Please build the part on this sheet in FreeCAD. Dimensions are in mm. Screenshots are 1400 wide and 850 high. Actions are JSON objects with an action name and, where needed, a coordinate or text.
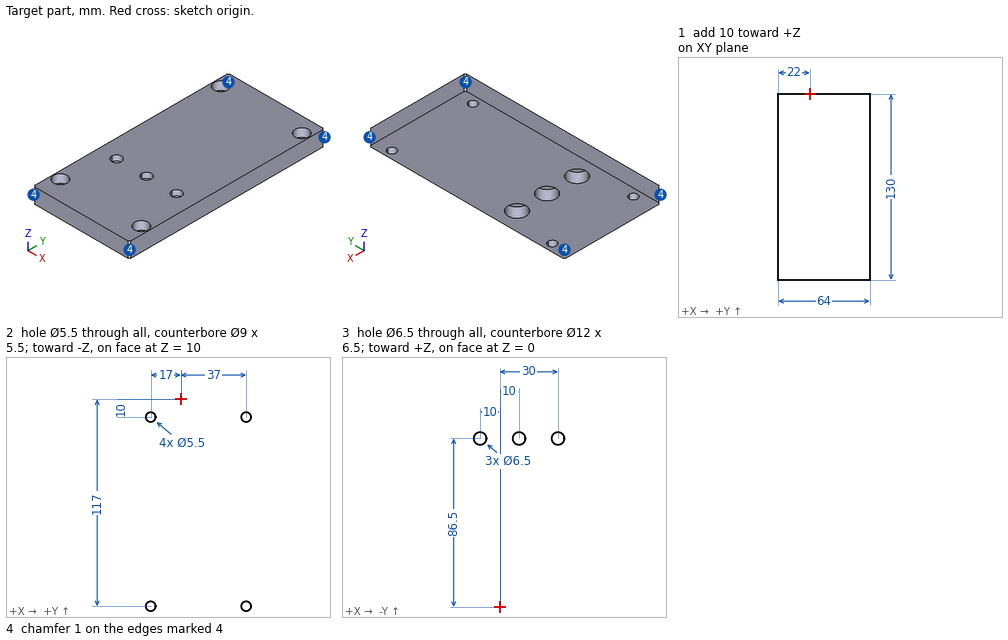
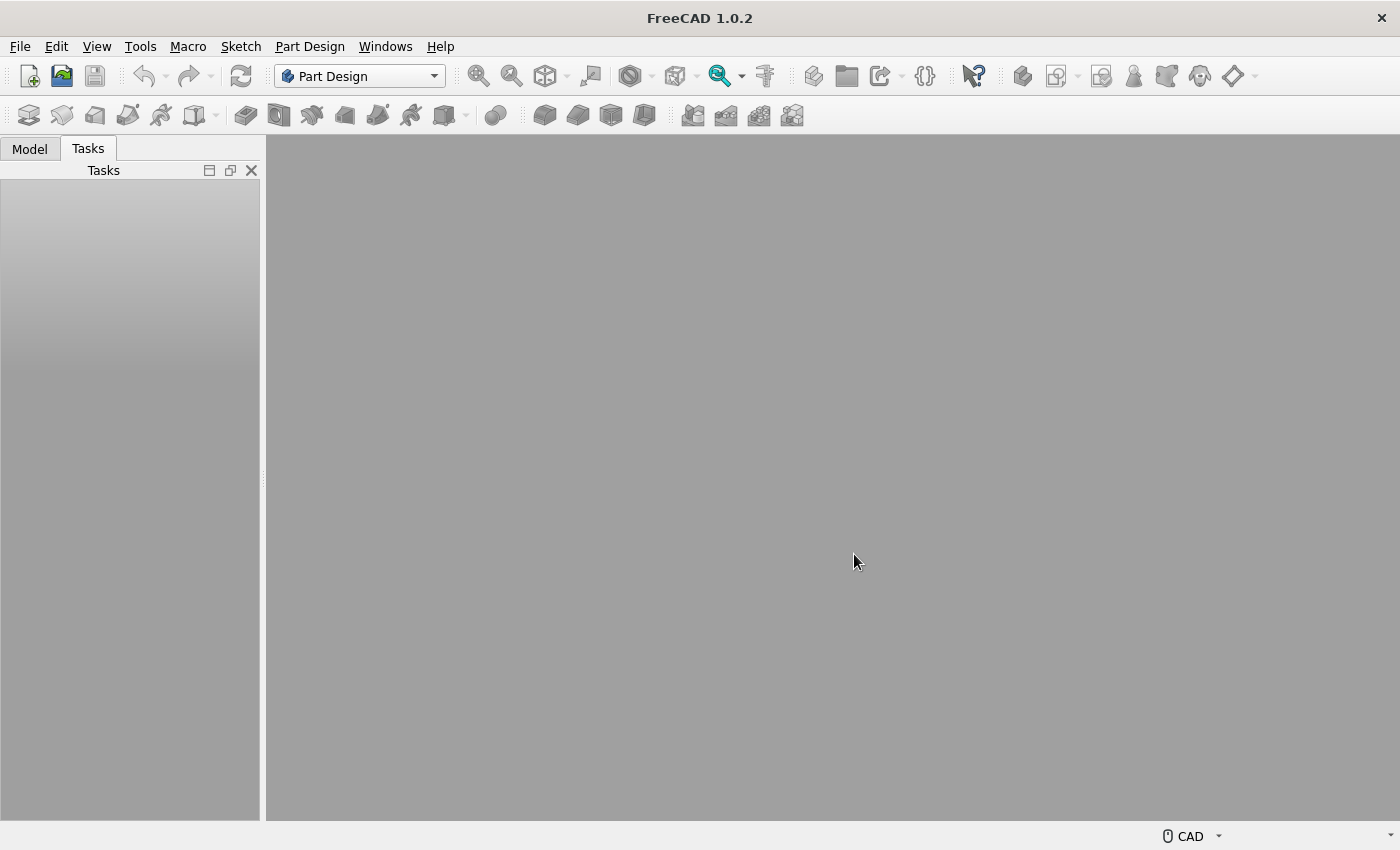
{"action": "left_click", "coordinate": [29, 76]}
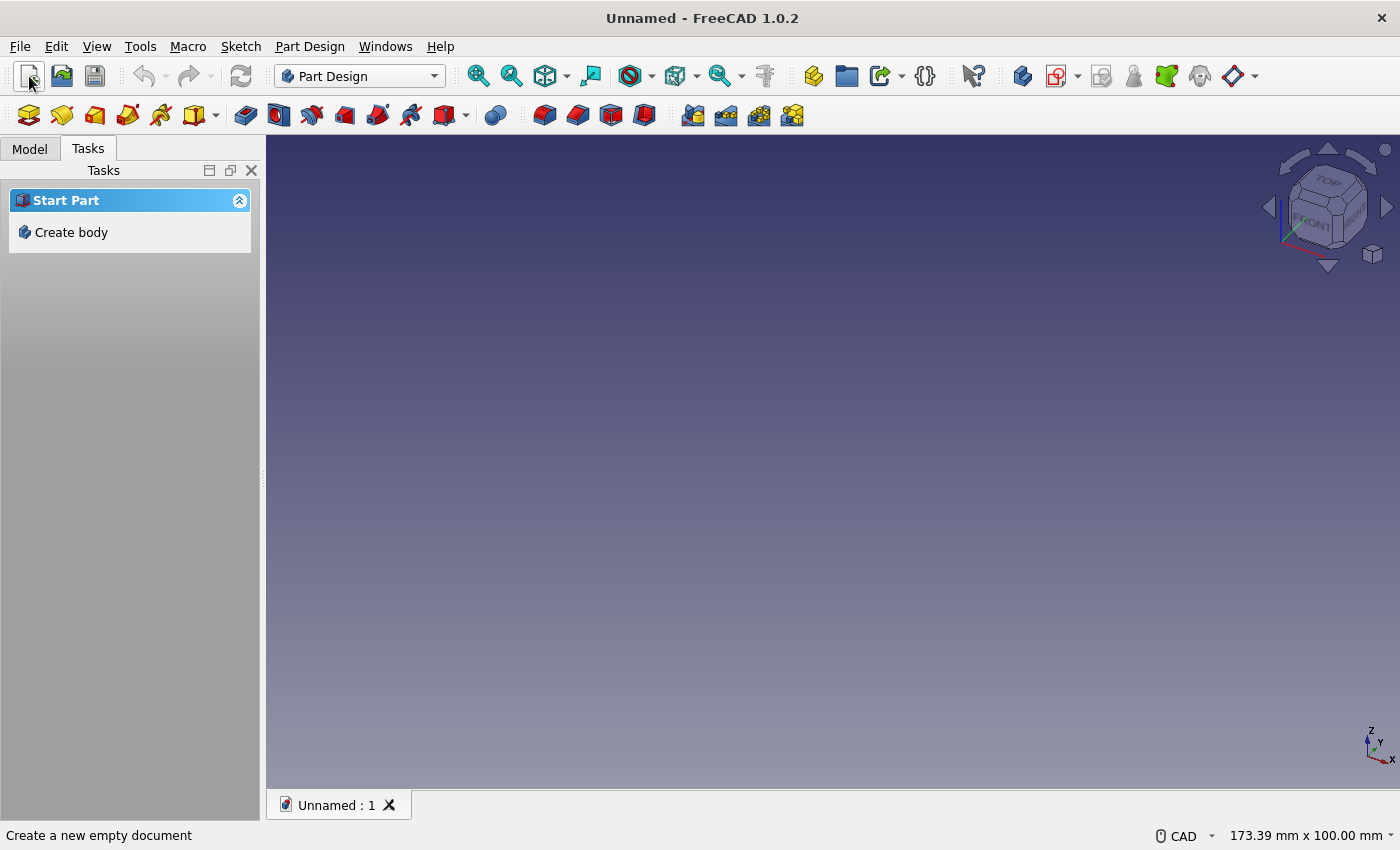
{"action": "left_click", "coordinate": [1056, 76]}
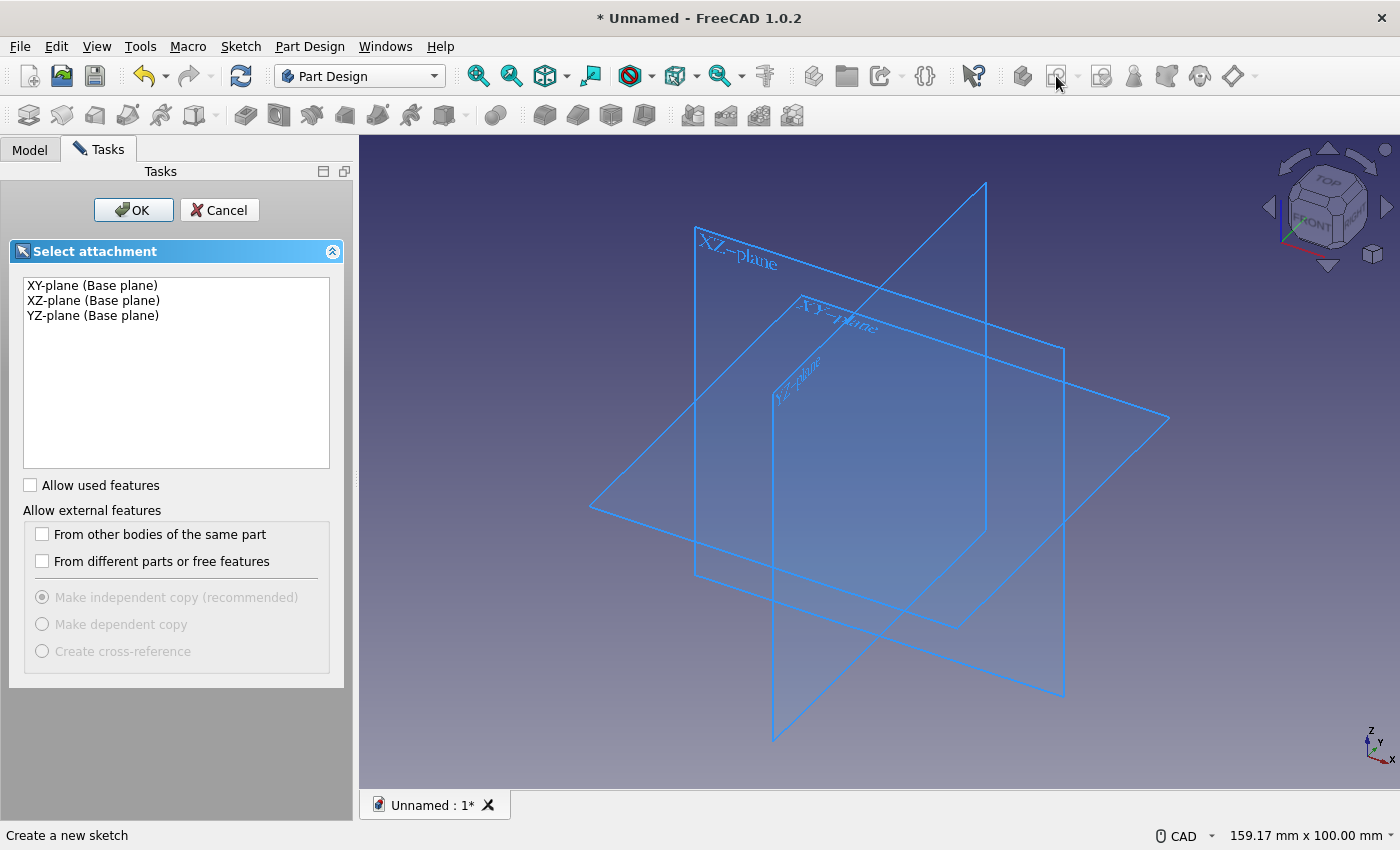
{"action": "left_click", "coordinate": [84, 286]}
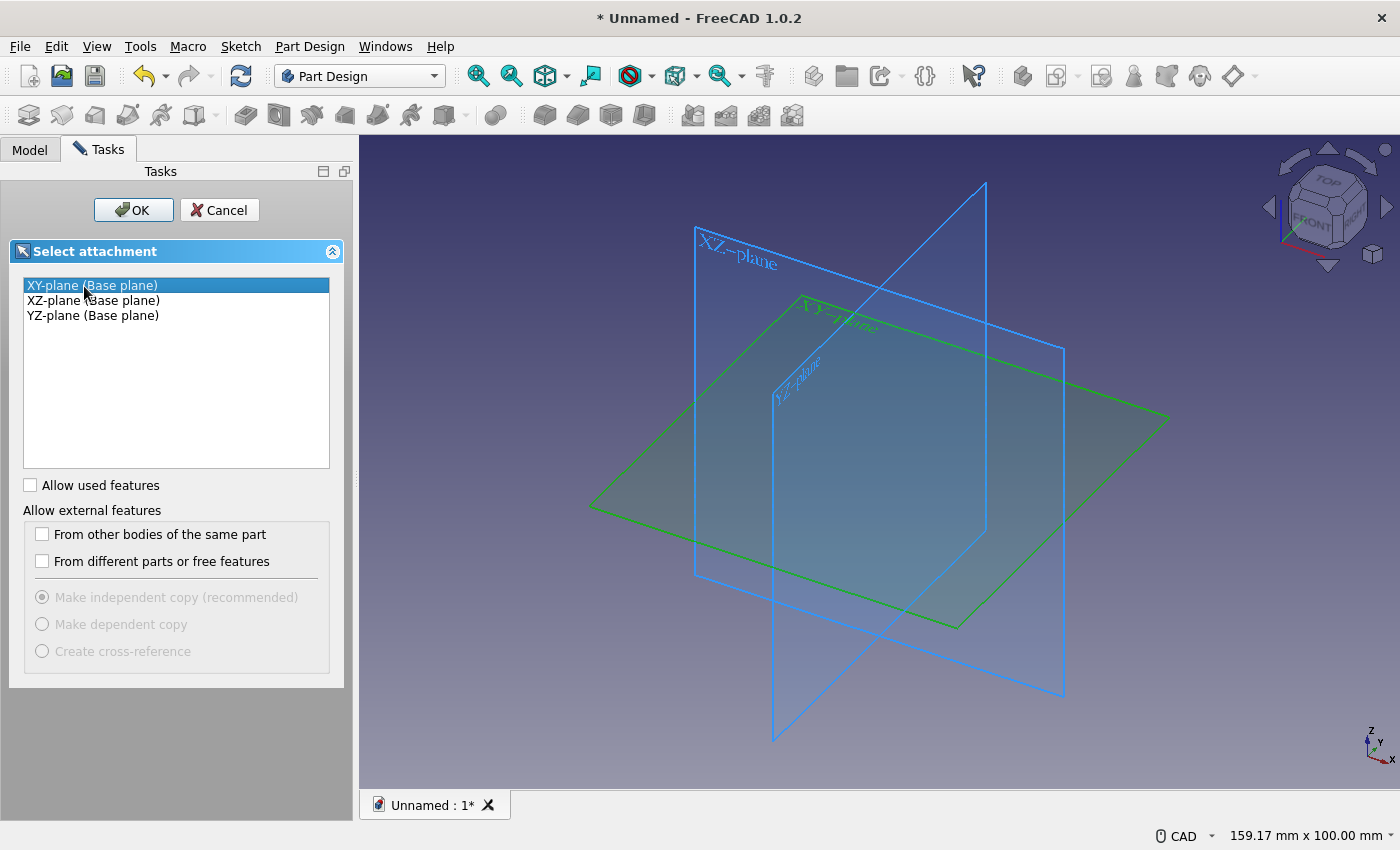
{"action": "left_click", "coordinate": [134, 210]}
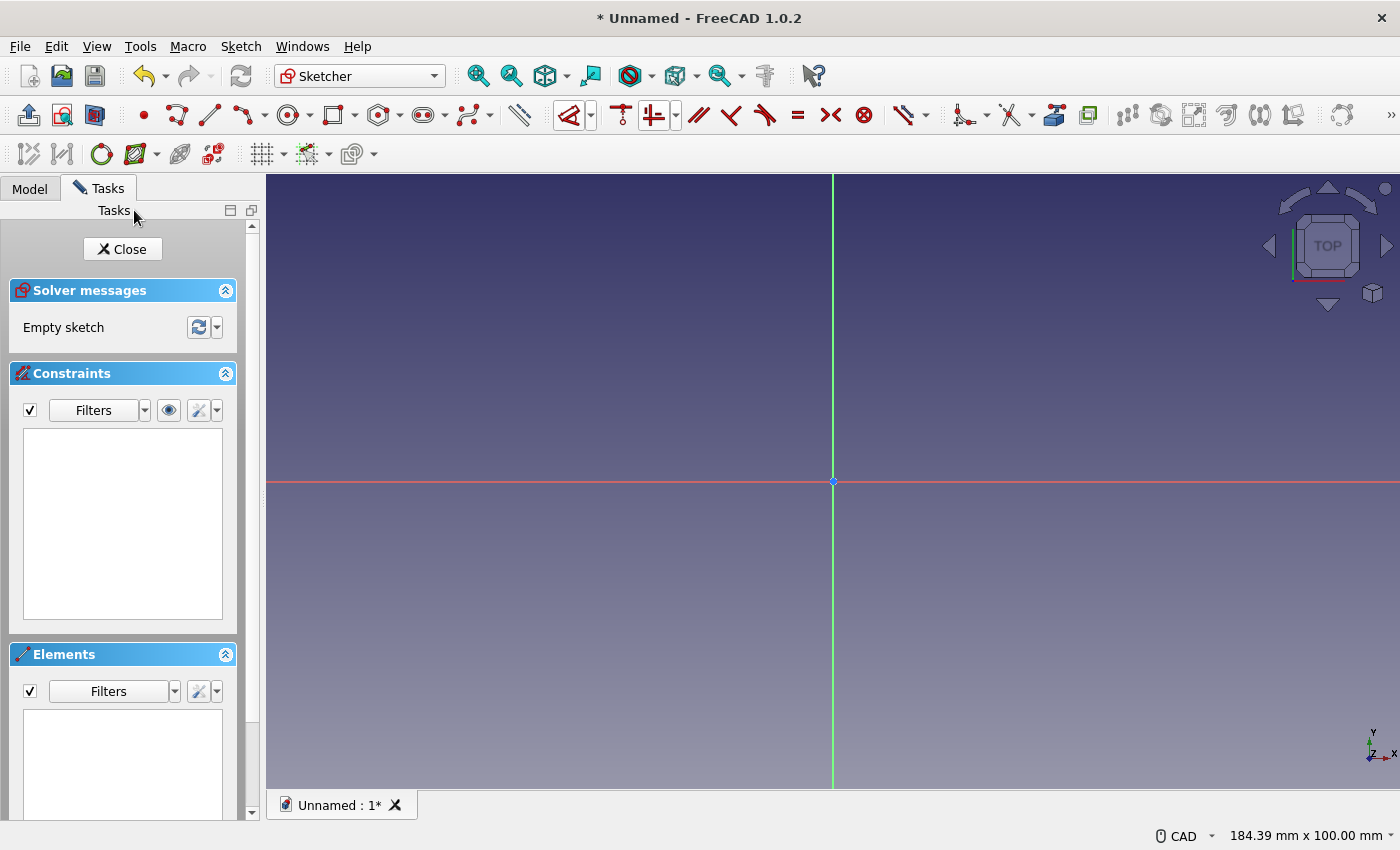
{"action": "scroll", "coordinate": [658, 202], "scroll_direction": "down", "scroll_amount": 4}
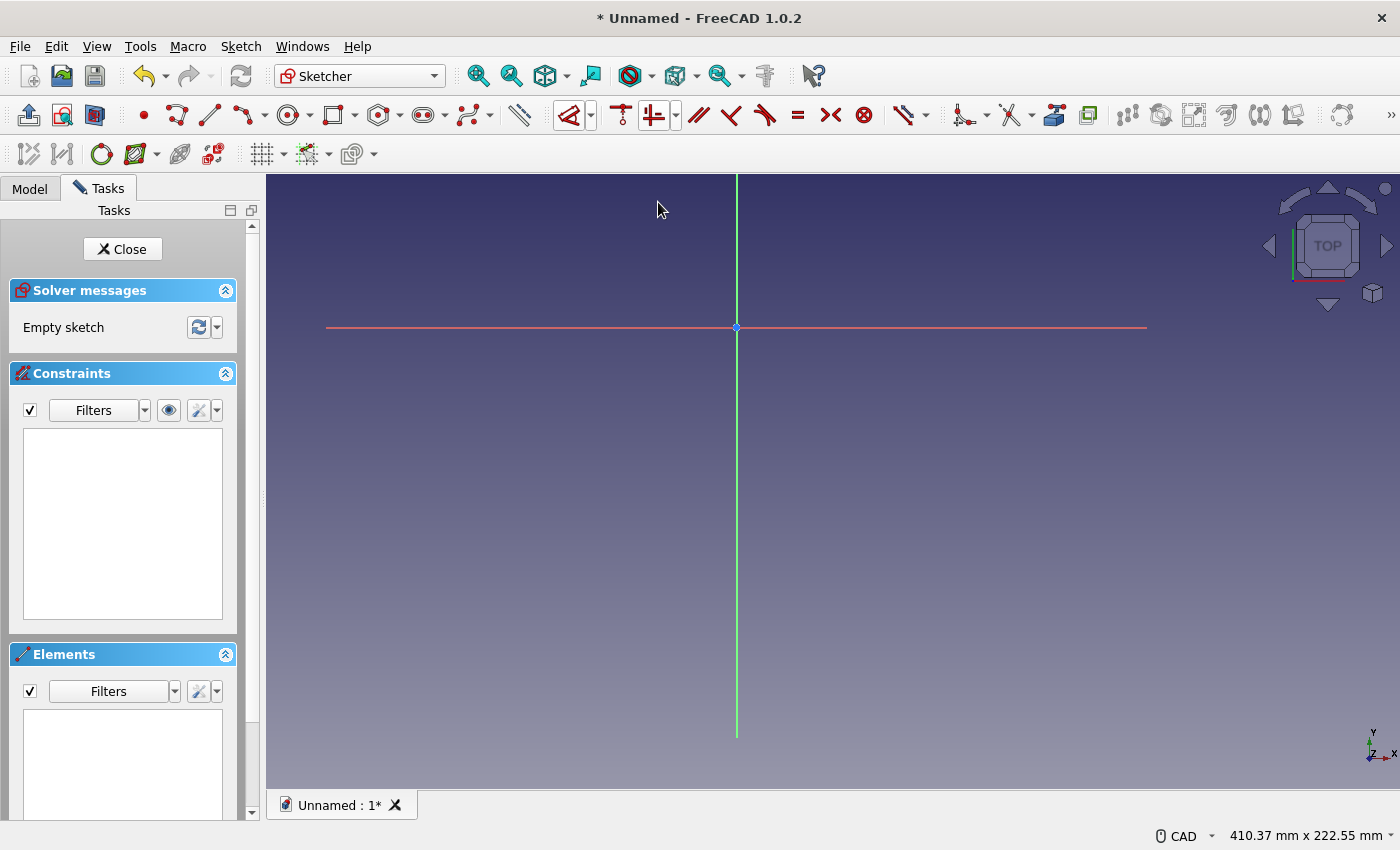
{"action": "left_click", "coordinate": [332, 116]}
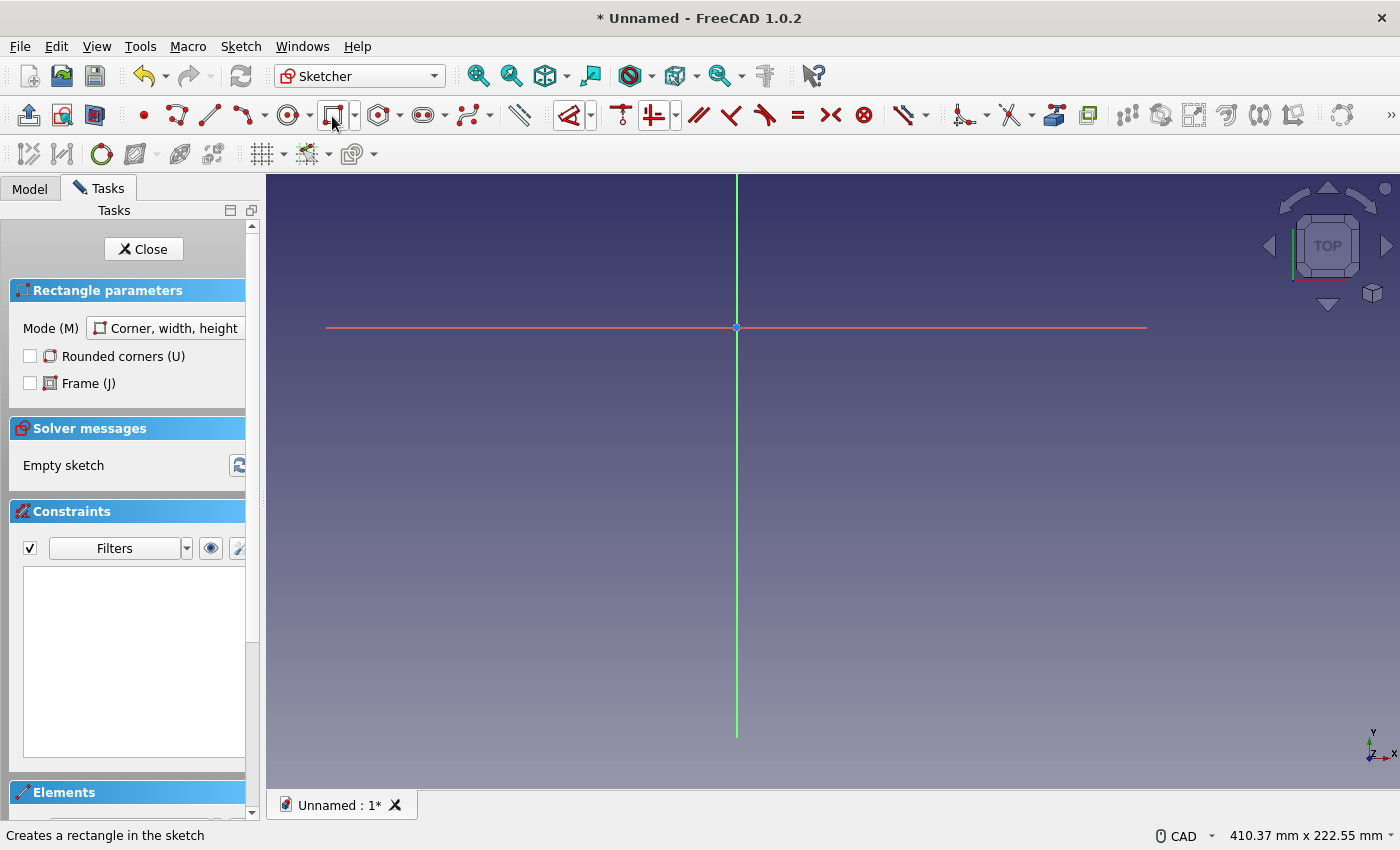
{"action": "left_click", "coordinate": [676, 328]}
{"action": "mouse_move", "coordinate": [853, 687]}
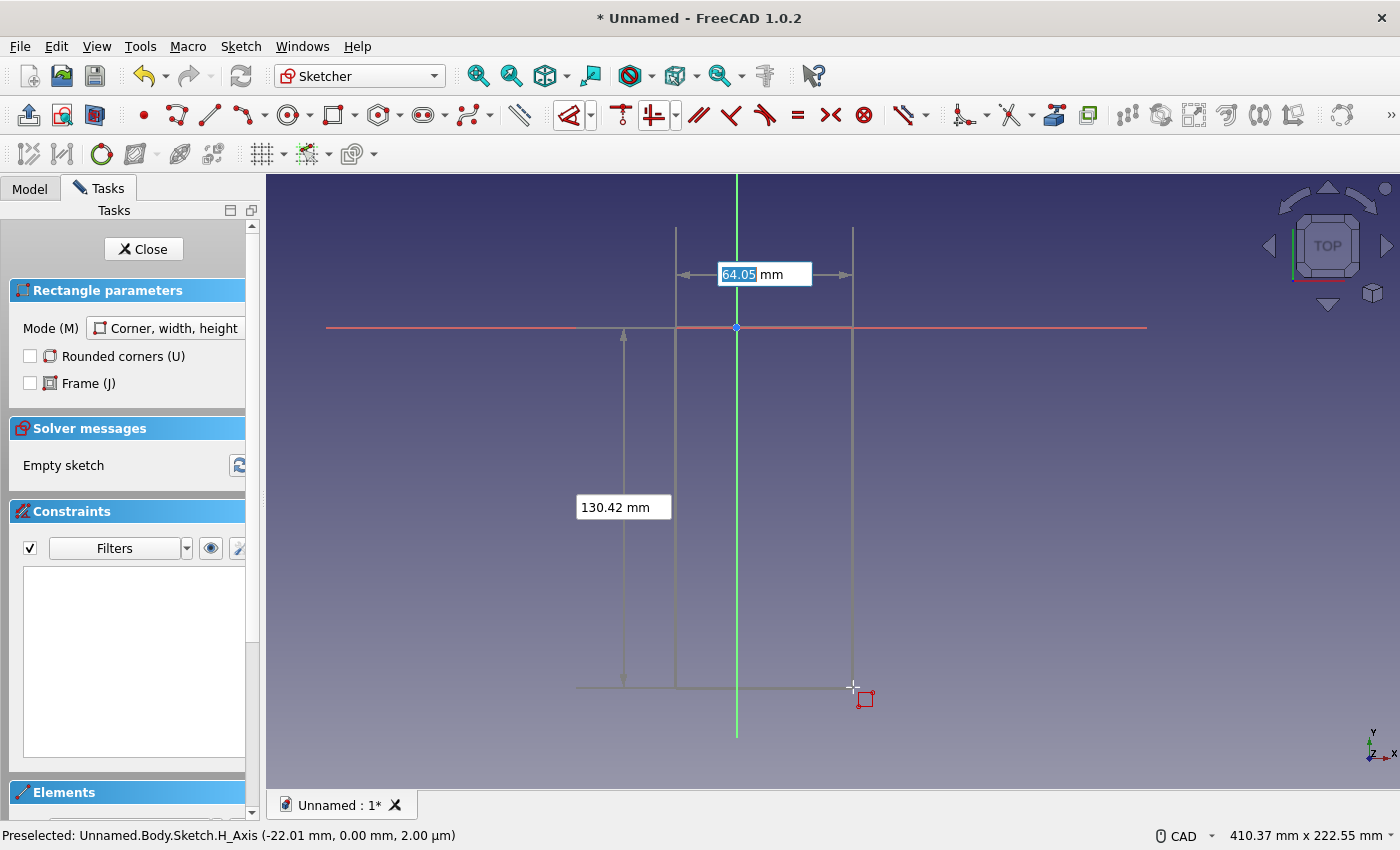
{"action": "type", "text": "64"}
{"action": "key", "text": "Tab"}
{"action": "type", "text": "130"}
{"action": "key", "text": "Return"}
{"action": "key", "text": "Escape"}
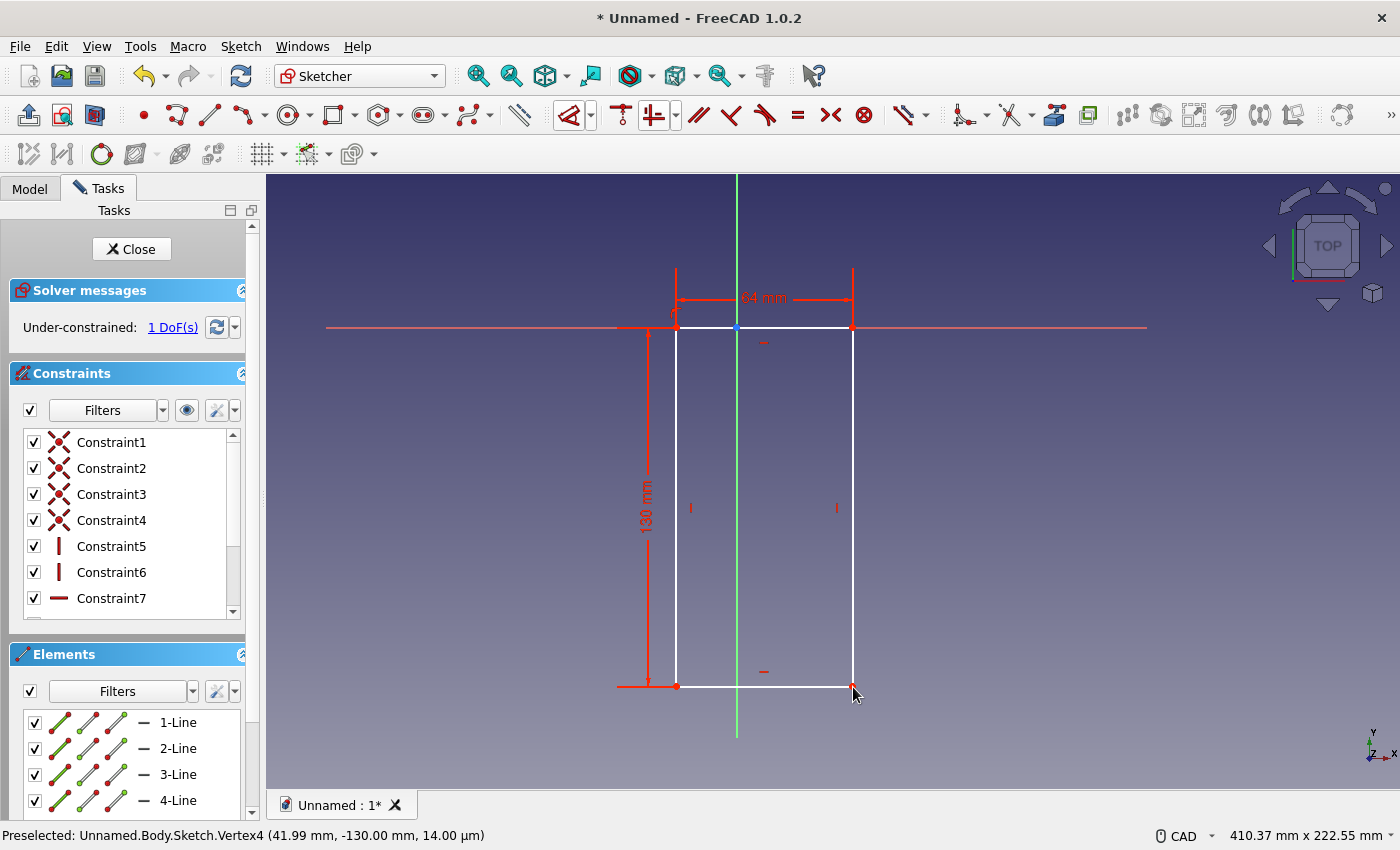
{"action": "left_click", "coordinate": [676, 328]}